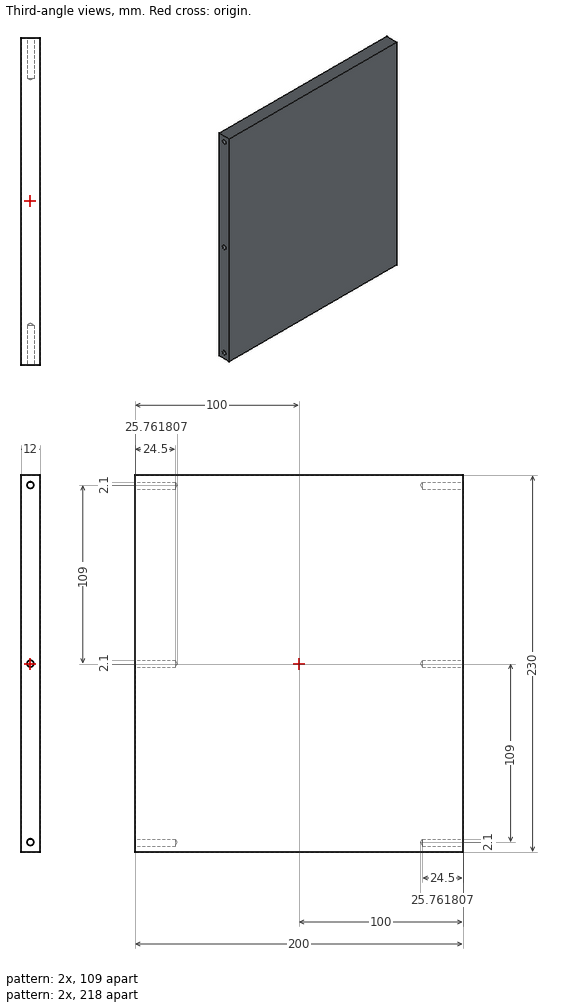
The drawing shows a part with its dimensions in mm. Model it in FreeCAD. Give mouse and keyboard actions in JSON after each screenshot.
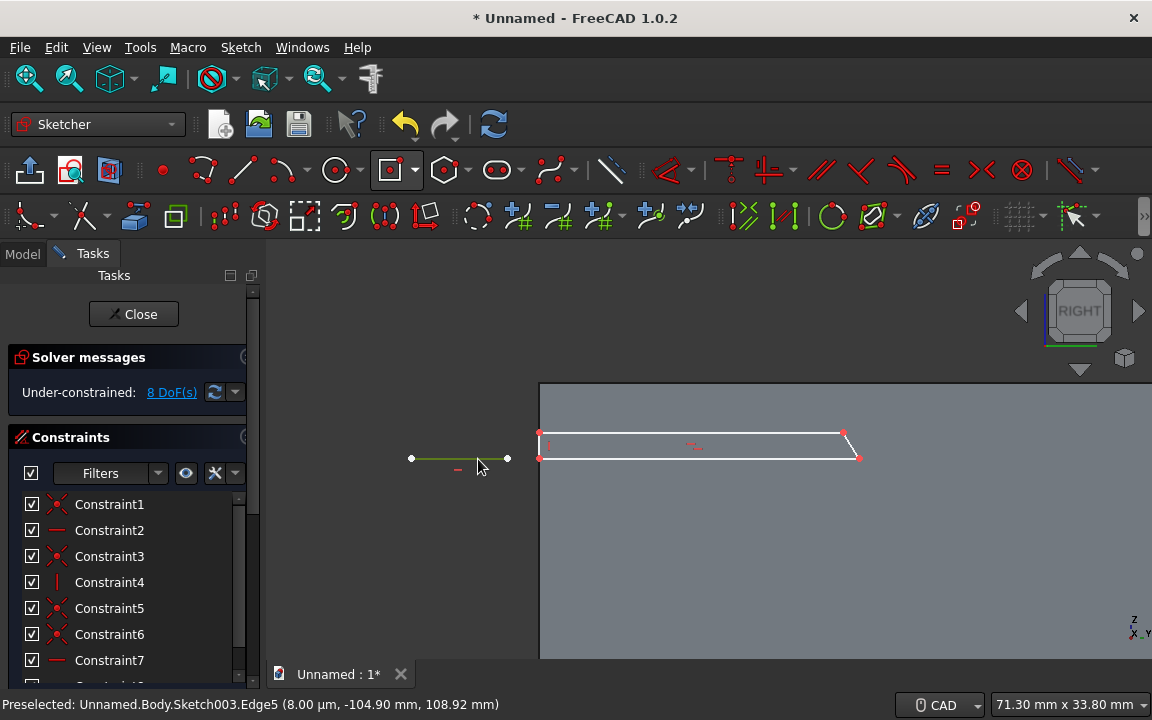
{"action": "left_click", "coordinate": [612, 170]}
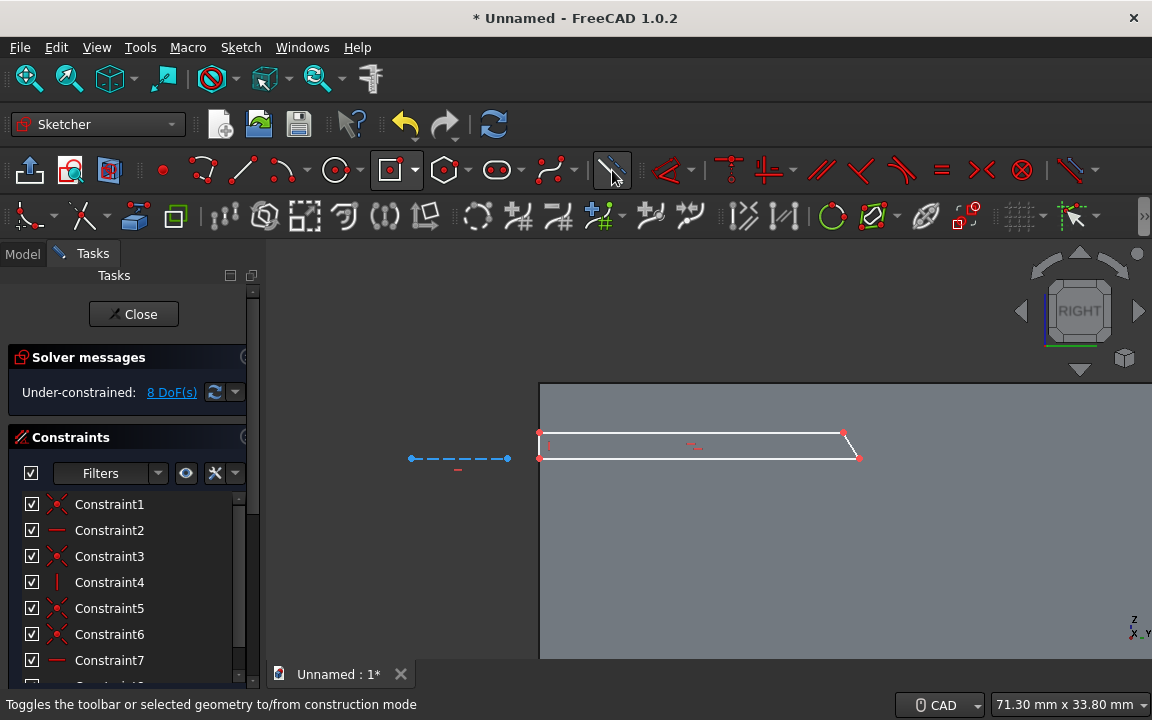
{"action": "left_click", "coordinate": [666, 170]}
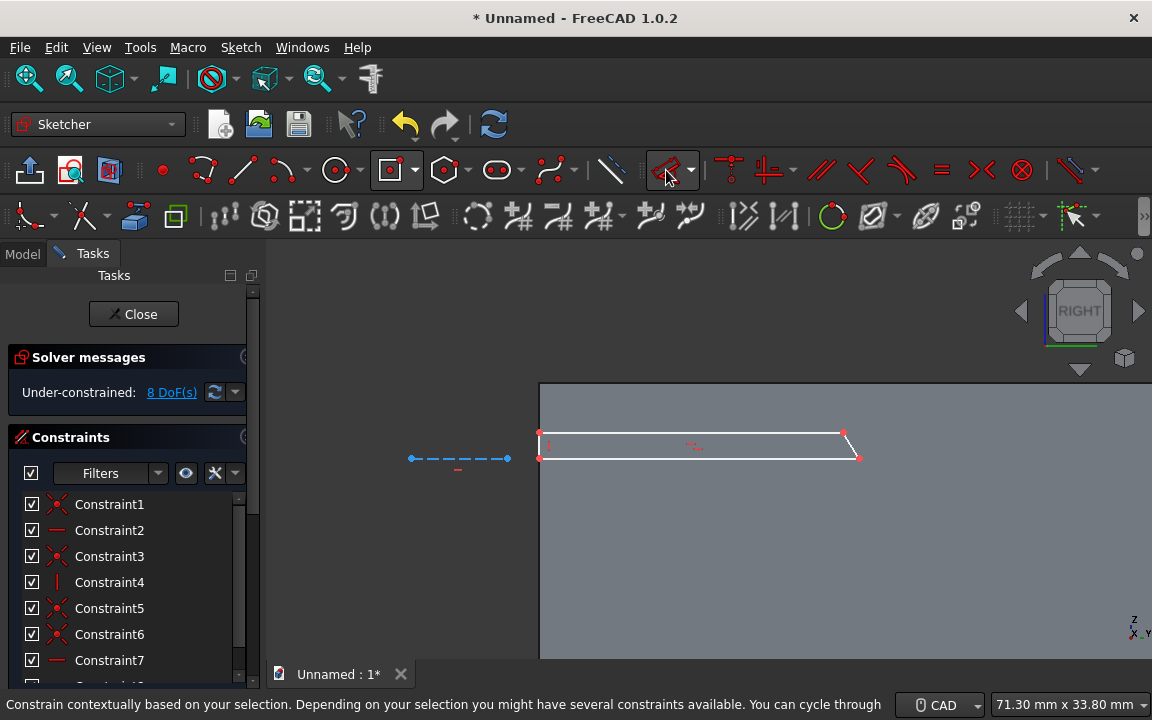
{"action": "scroll", "coordinate": [539, 443], "scroll_direction": "up", "scroll_amount": 3}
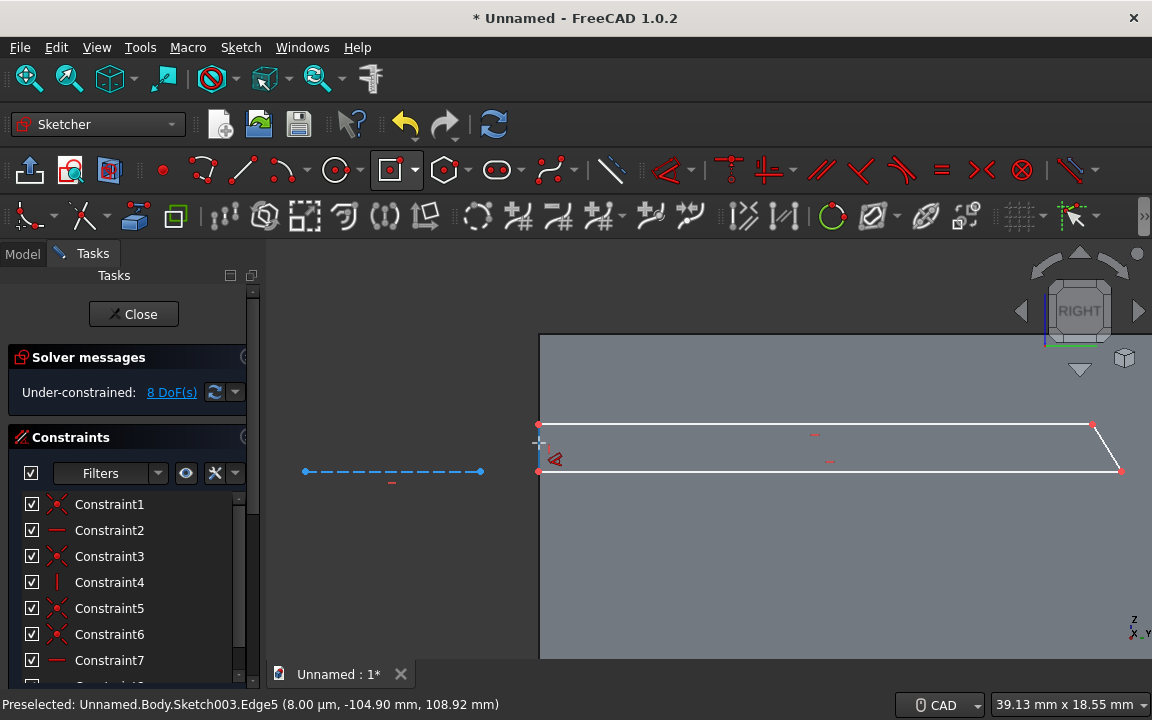
{"action": "left_click", "coordinate": [539, 443]}
{"action": "left_click", "coordinate": [505, 448]}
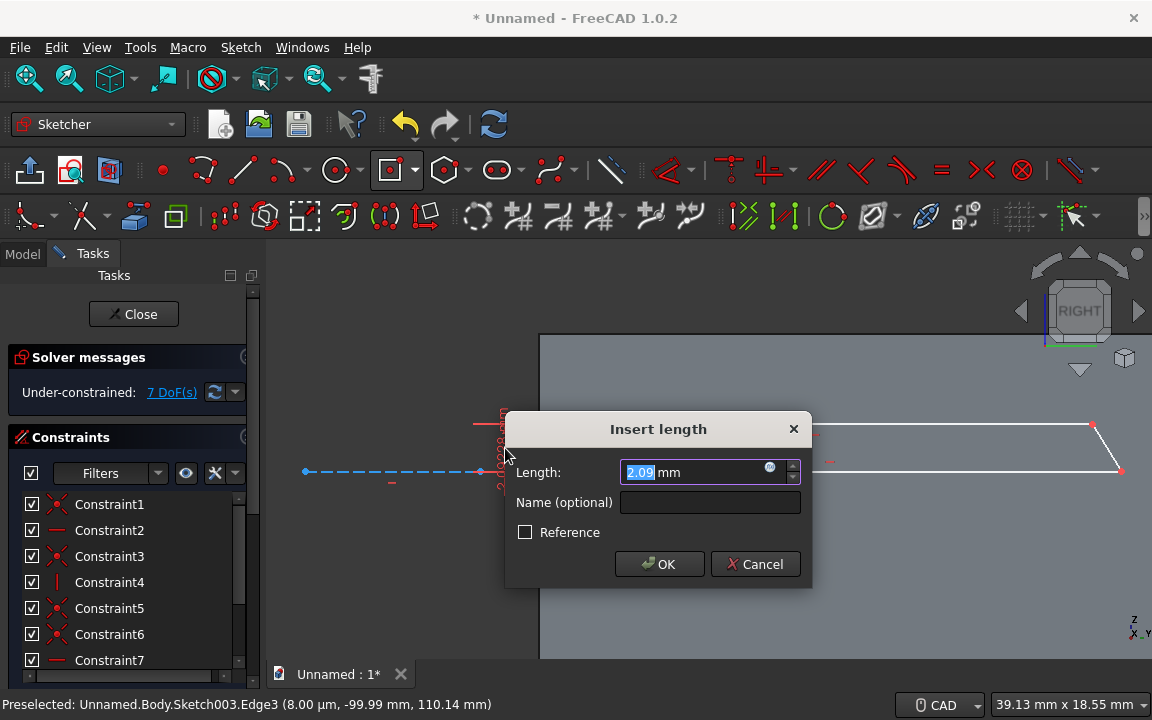
{"action": "type", "text": "2.1"}
{"action": "key", "text": "Return"}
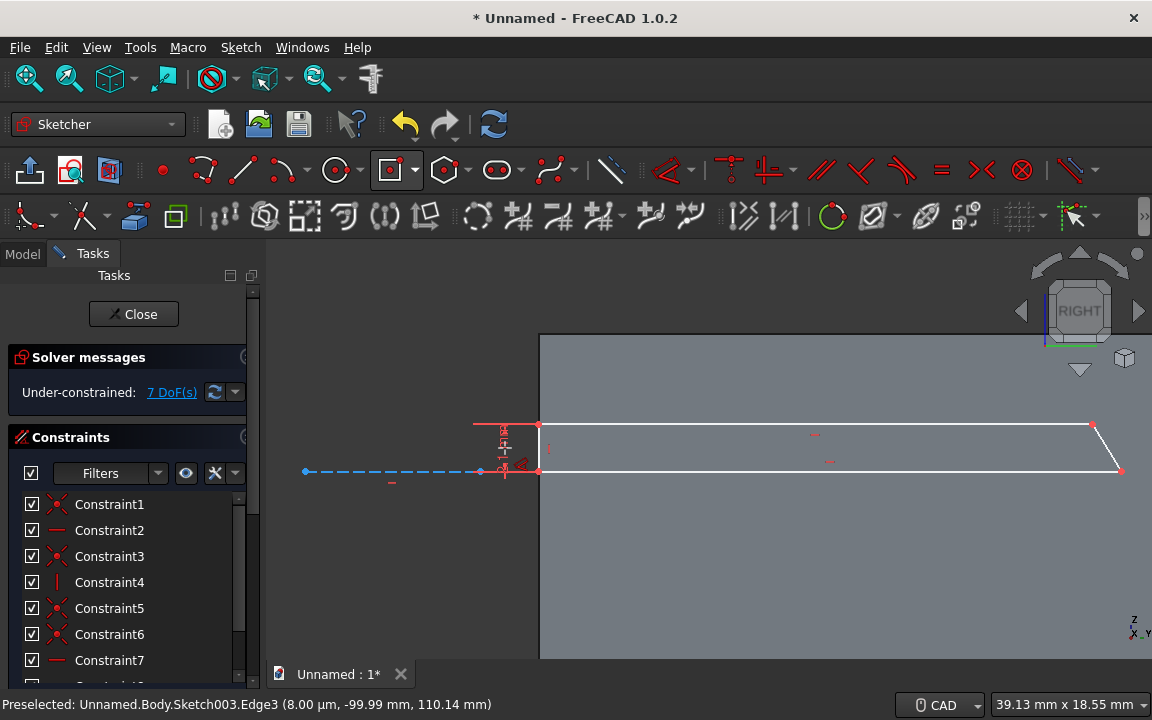
{"action": "left_click", "coordinate": [926, 424]}
{"action": "left_click", "coordinate": [763, 390]}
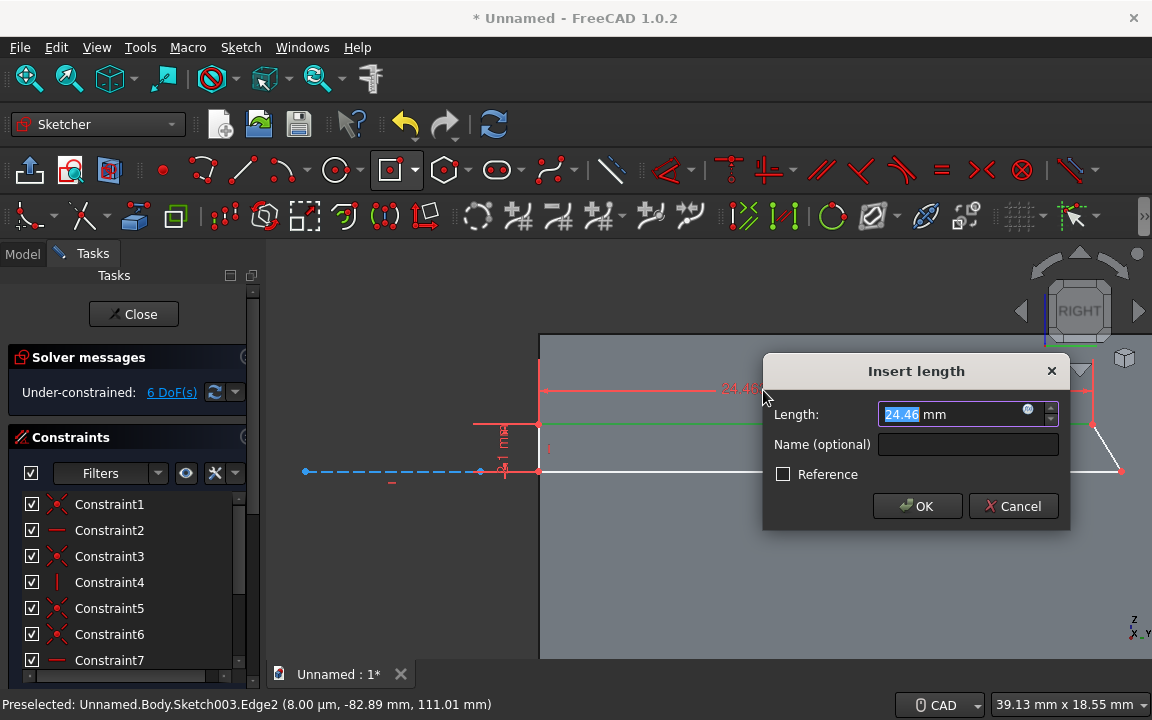
{"action": "type", "text": "24.5"}
{"action": "key", "text": "Return"}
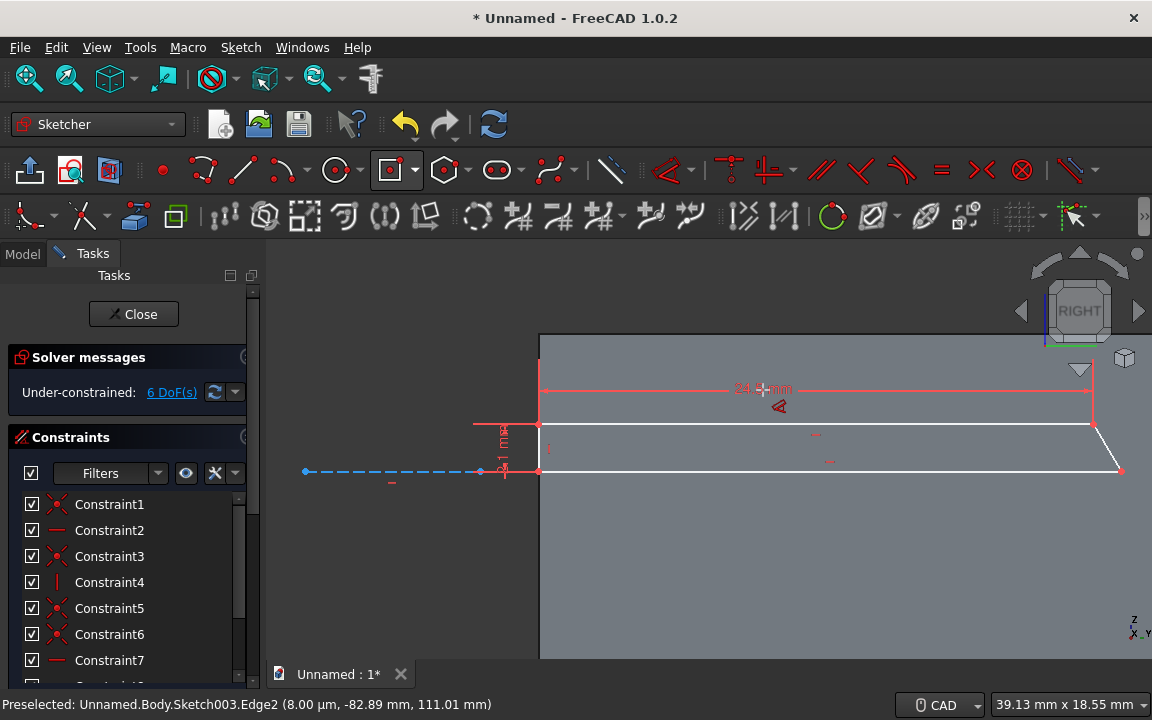
{"action": "scroll", "coordinate": [552, 452], "scroll_direction": "down", "scroll_amount": 3}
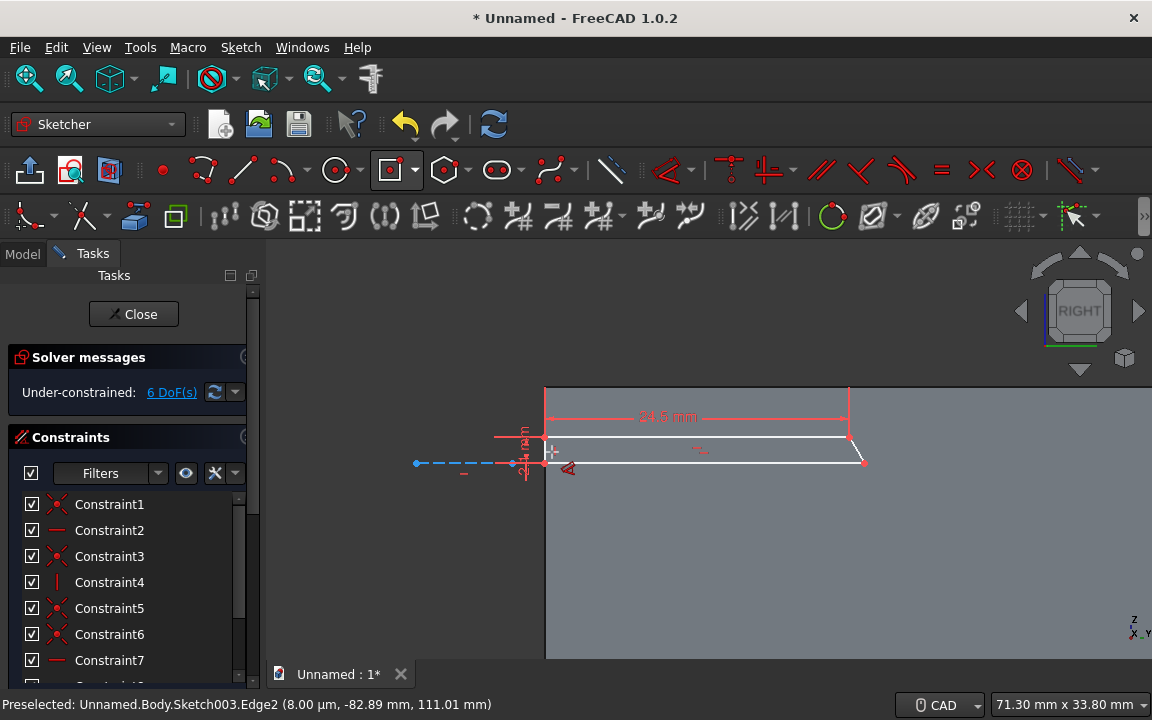
{"action": "left_click", "coordinate": [865, 463]}
{"action": "left_click", "coordinate": [831, 547]}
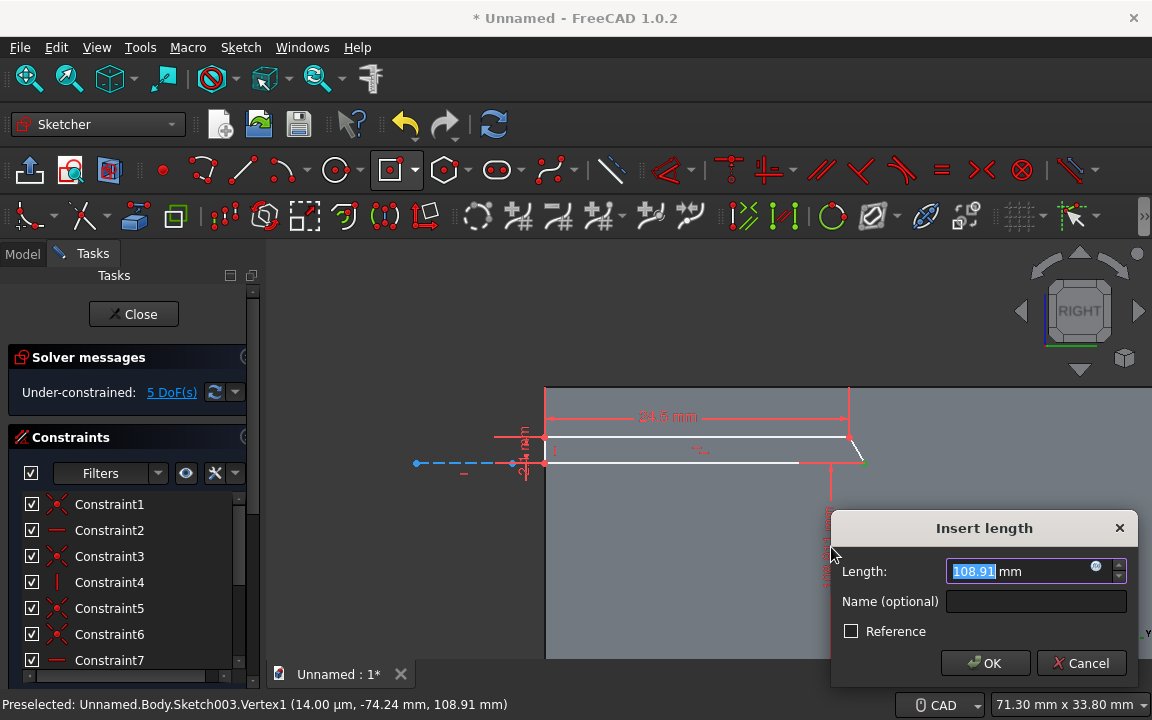
{"action": "type", "text": "109"}
{"action": "key", "text": "Return"}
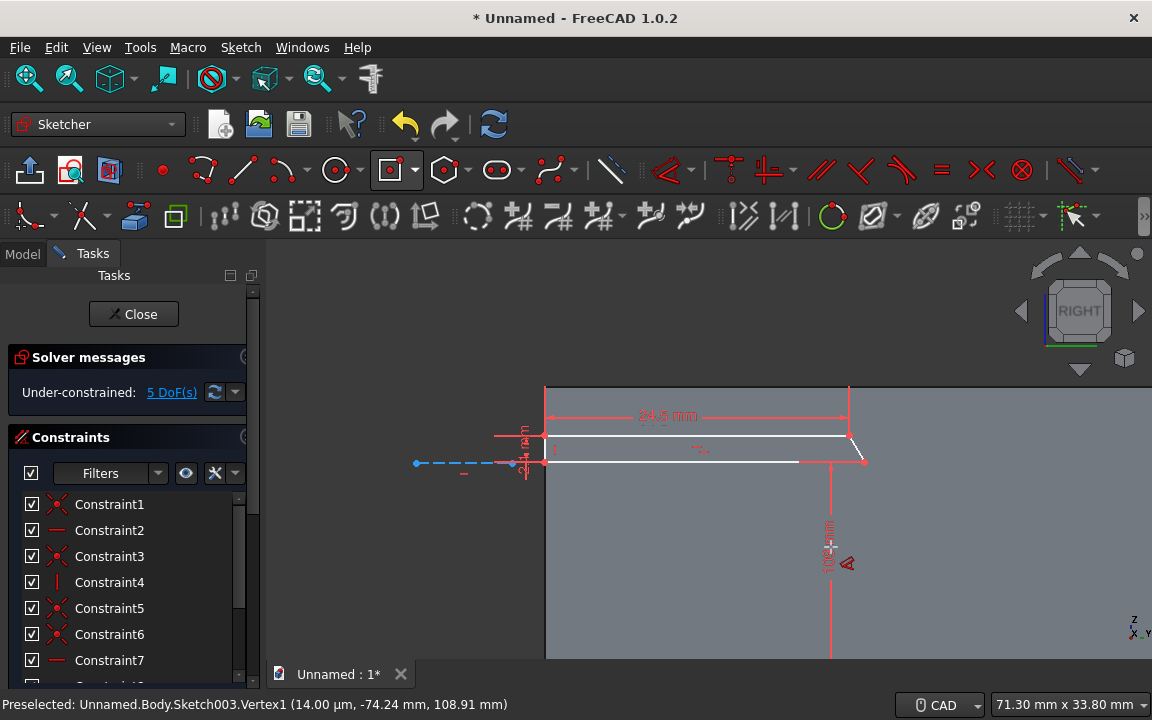
{"action": "left_click", "coordinate": [545, 436]}
{"action": "left_click", "coordinate": [766, 402]}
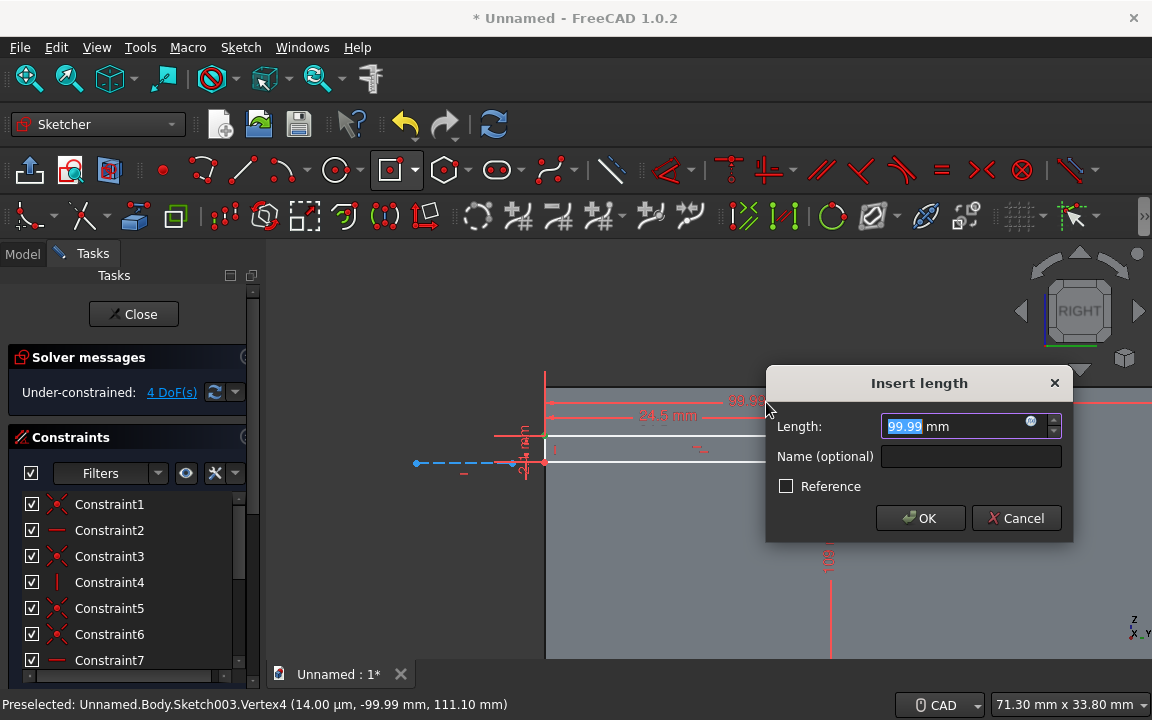
{"action": "type", "text": "100"}
{"action": "key", "text": "Return"}